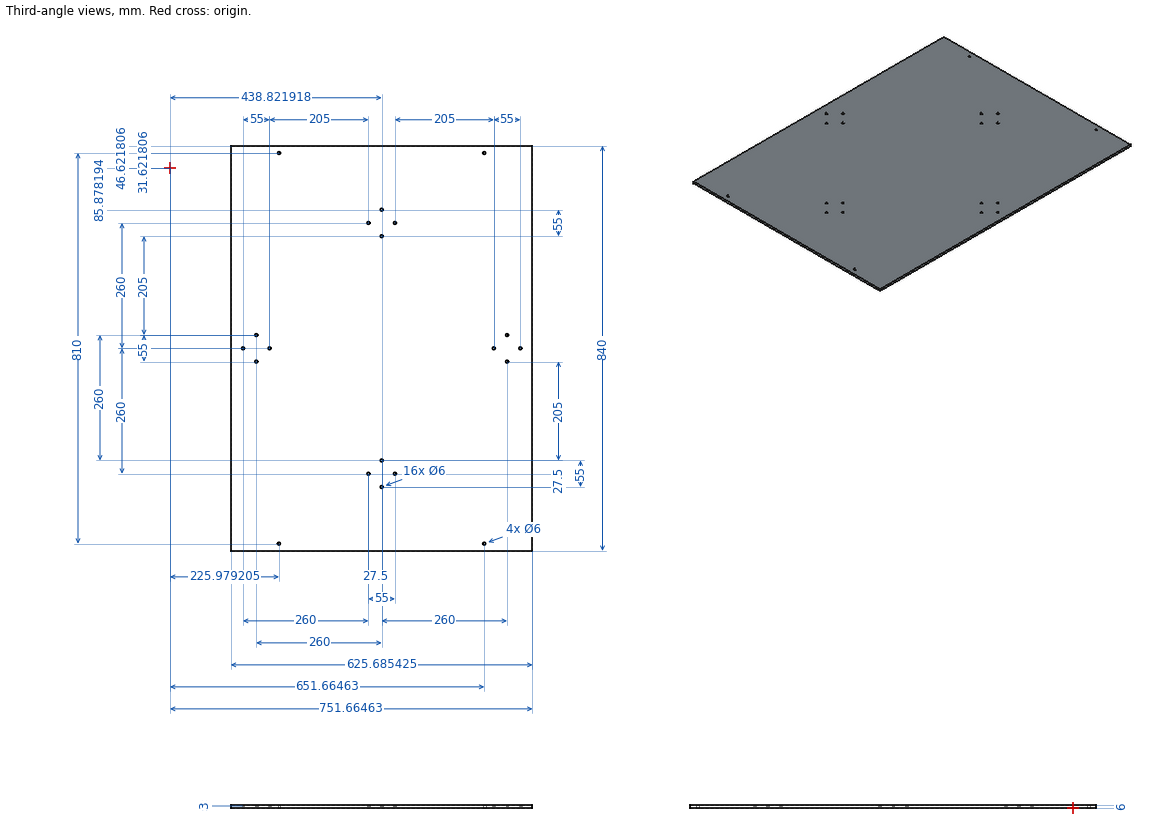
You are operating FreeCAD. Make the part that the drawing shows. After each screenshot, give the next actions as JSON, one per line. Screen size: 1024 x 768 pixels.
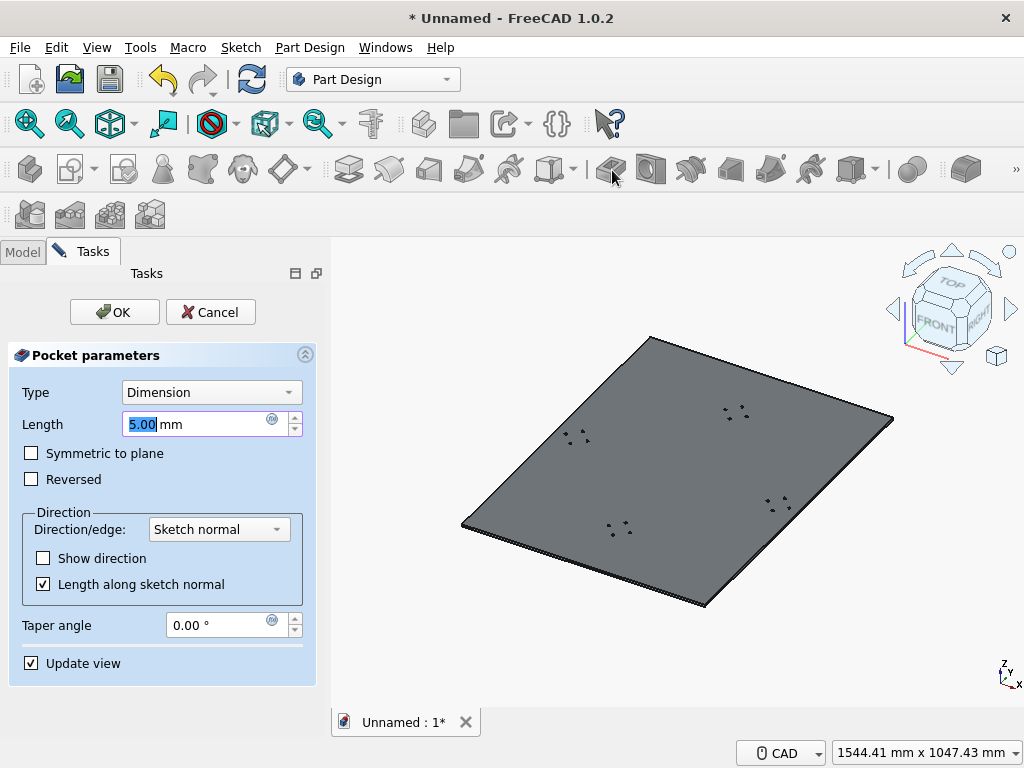
{"action": "type", "text": "3"}
{"action": "key", "text": "Tab"}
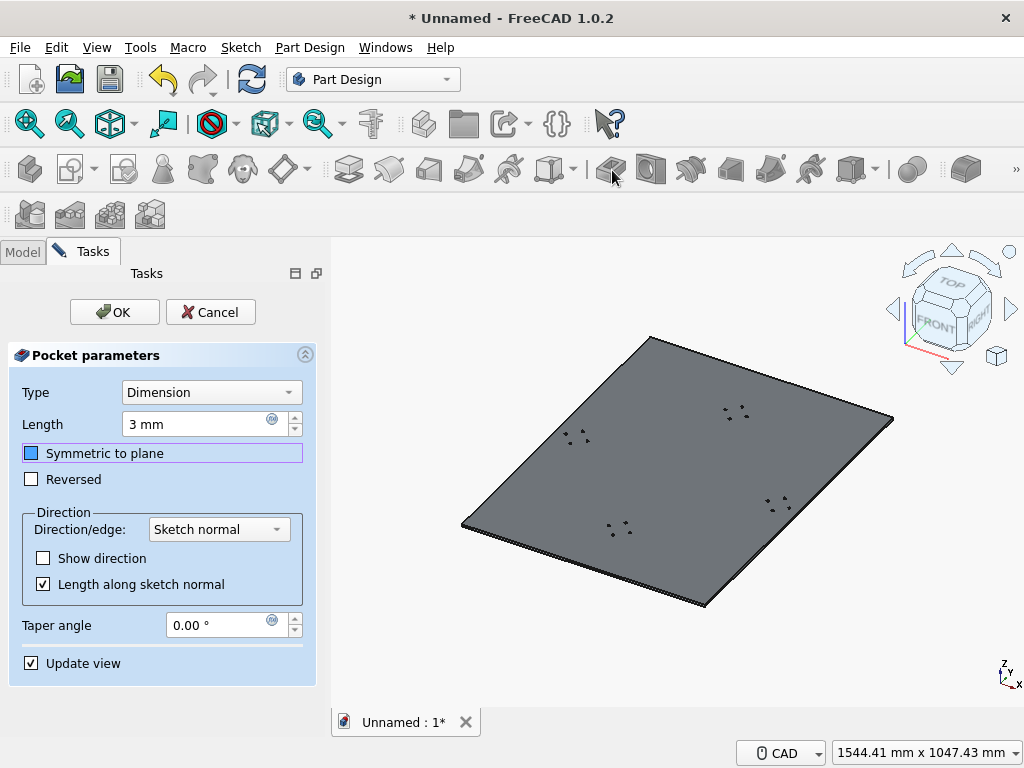
{"action": "left_click", "coordinate": [115, 312]}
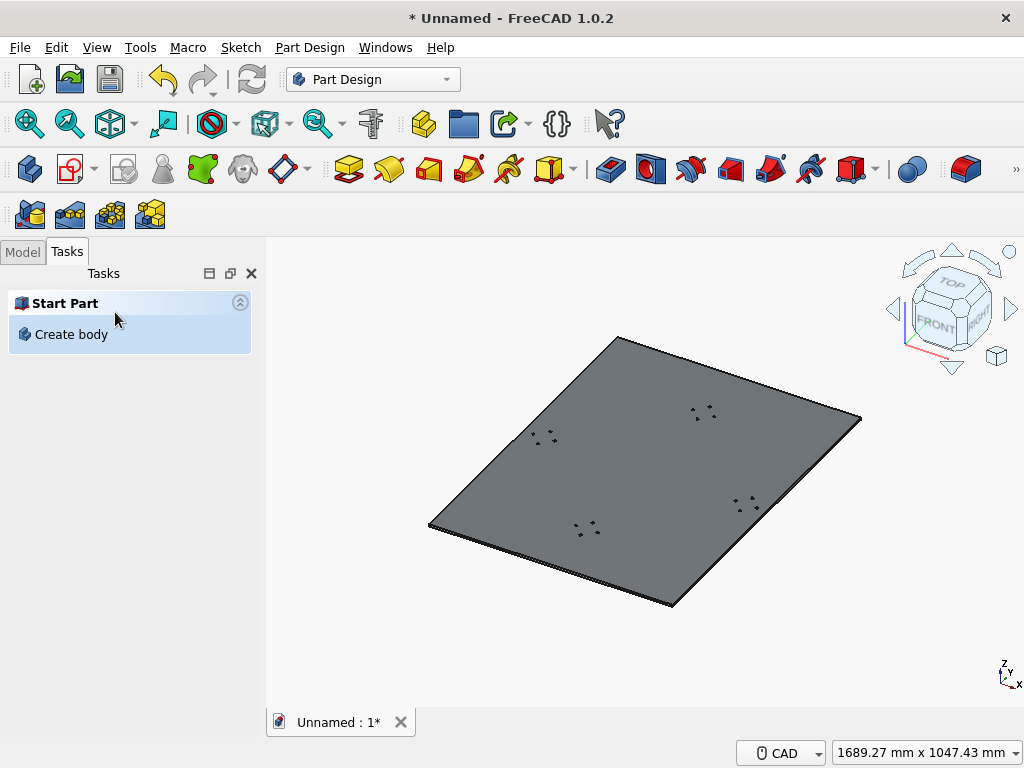
{"action": "left_click", "coordinate": [645, 470]}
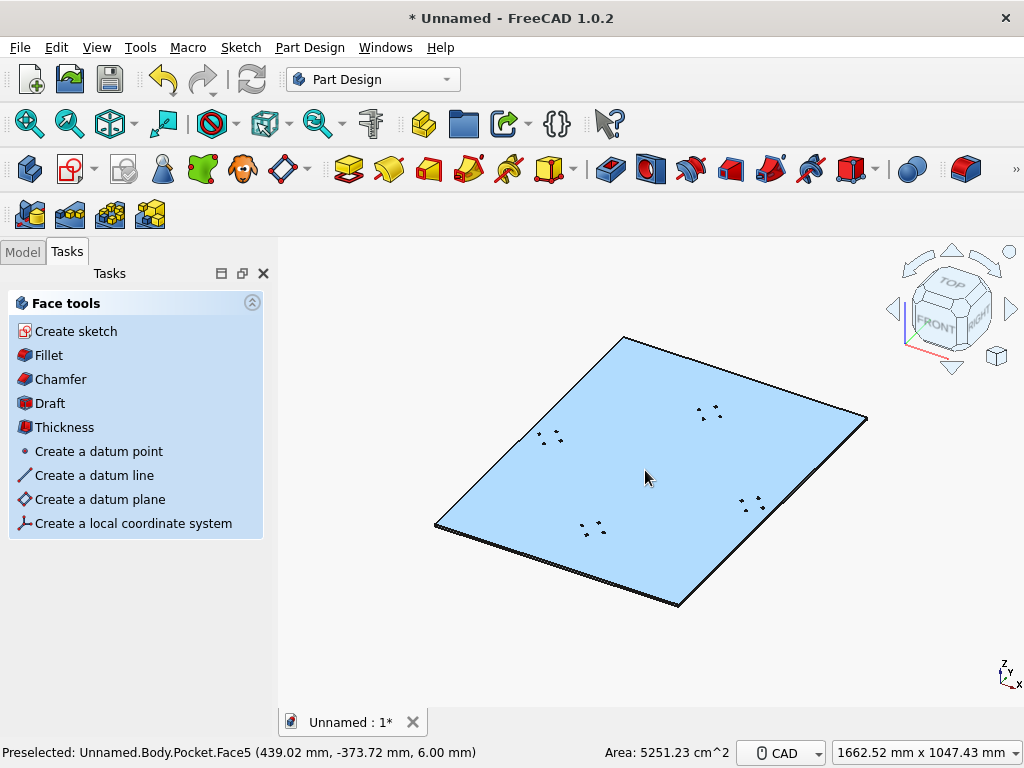
{"action": "left_click", "coordinate": [70, 170]}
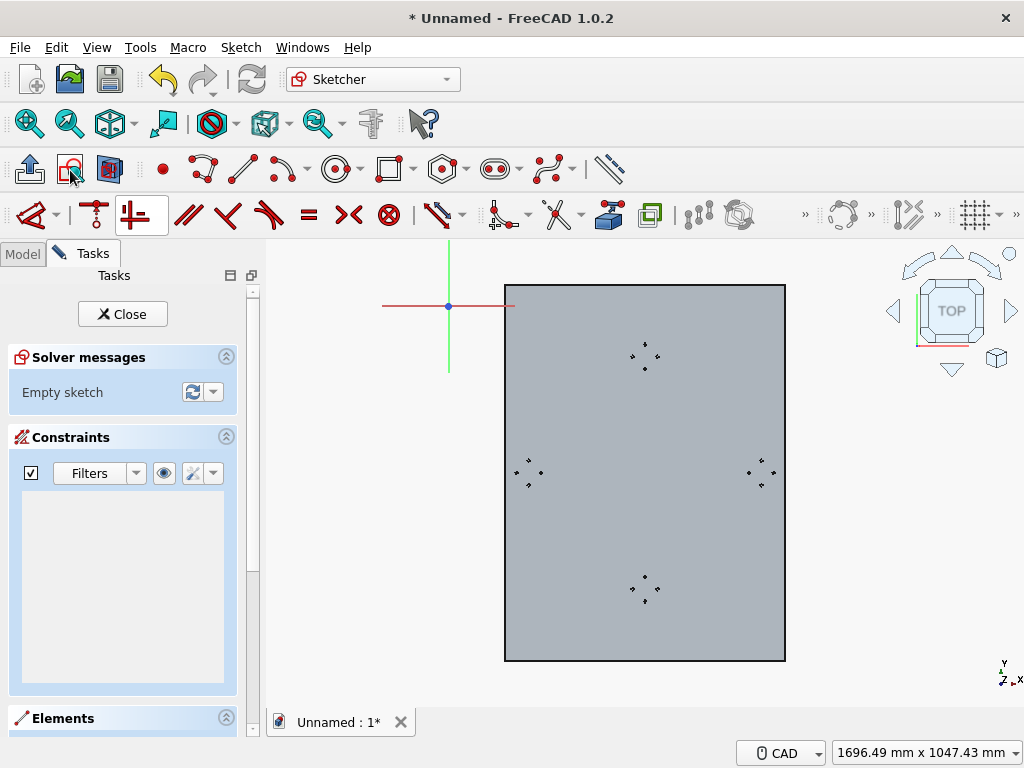
{"action": "scroll", "coordinate": [492, 473], "scroll_direction": "down", "scroll_amount": 1}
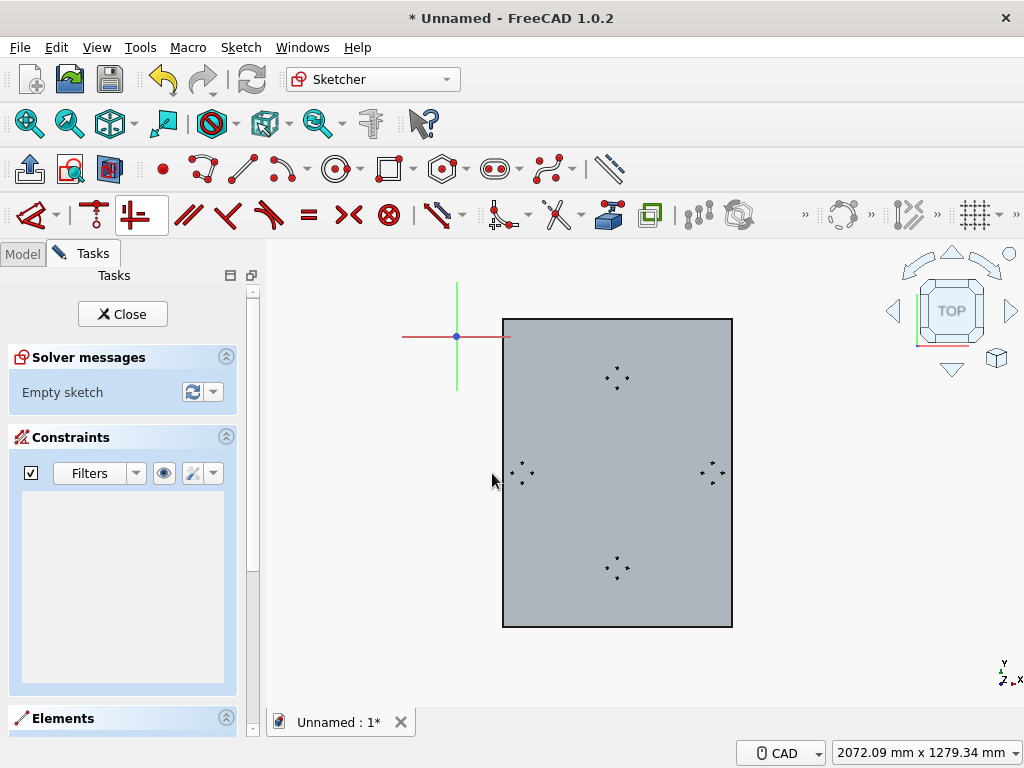
{"action": "left_click", "coordinate": [336, 170]}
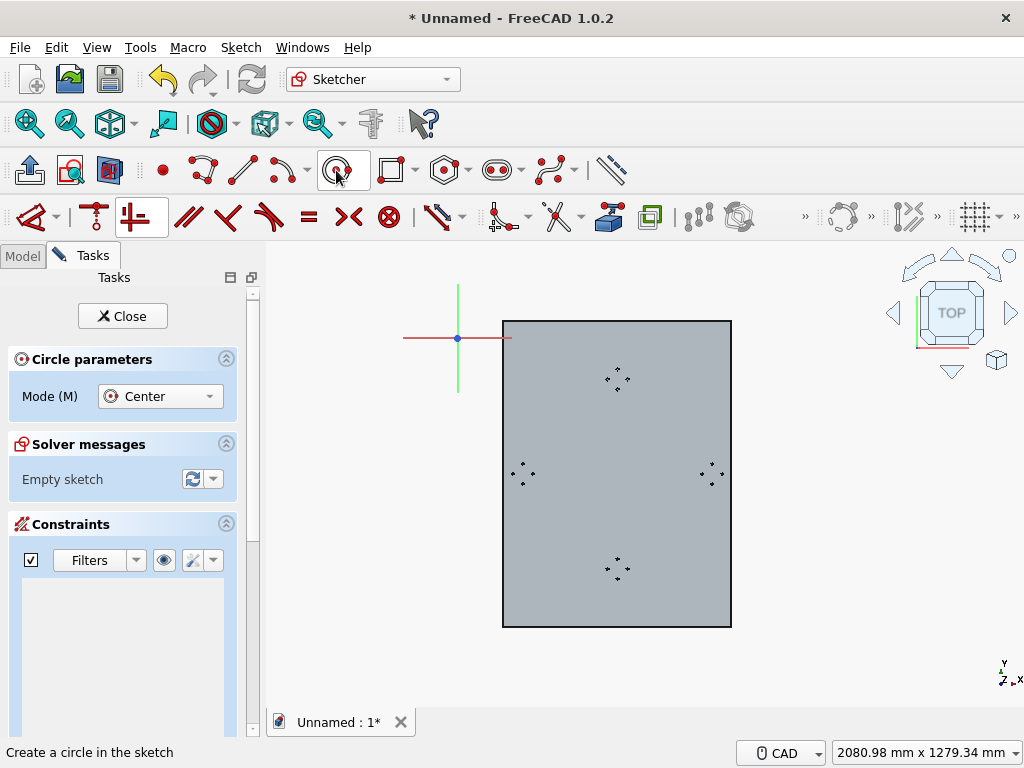
{"action": "scroll", "coordinate": [695, 622], "scroll_direction": "up", "scroll_amount": 16}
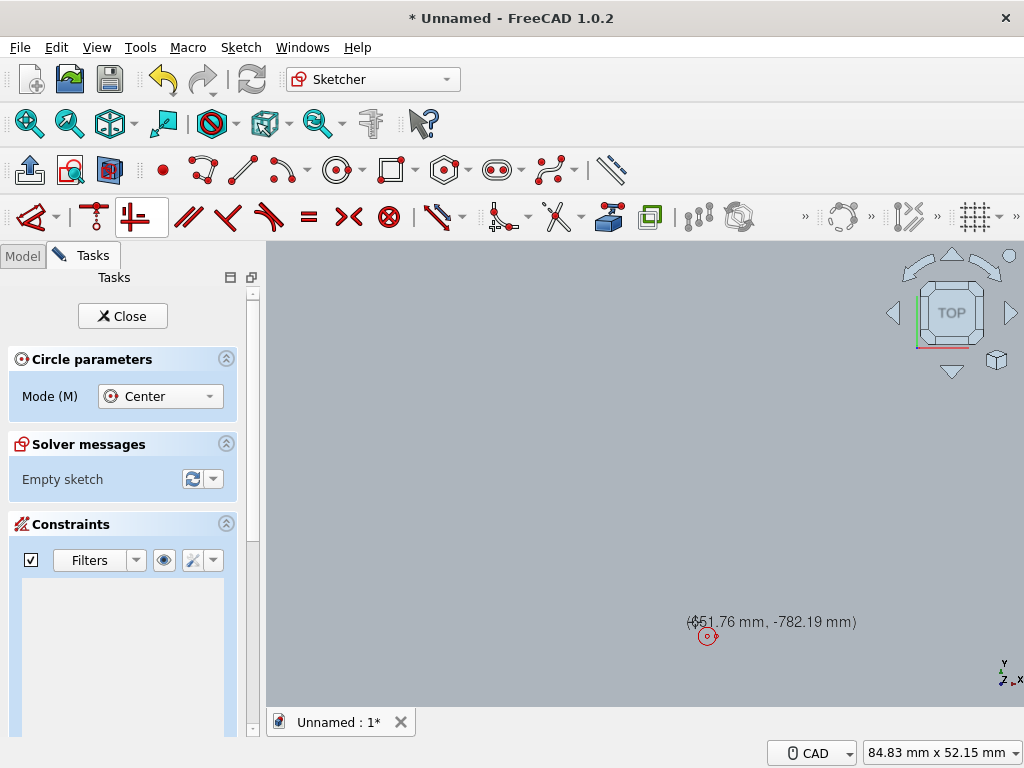
{"action": "scroll", "coordinate": [695, 623], "scroll_direction": "down", "scroll_amount": 16}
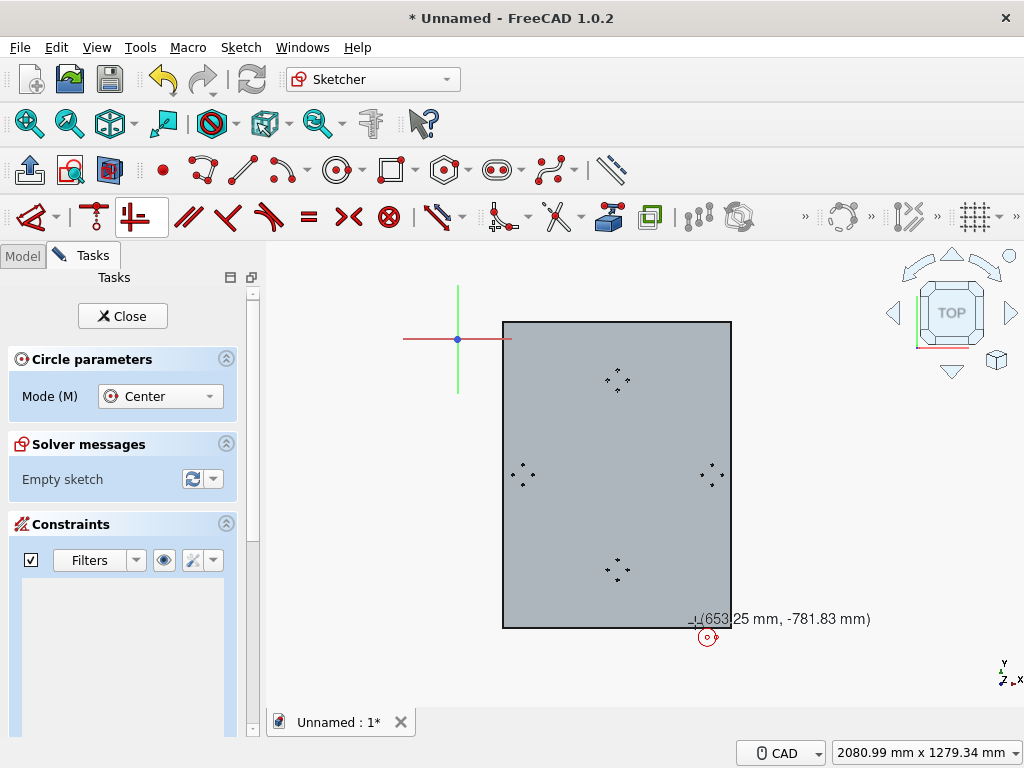
{"action": "left_click", "coordinate": [695, 623]}
{"action": "mouse_move", "coordinate": [696, 622]}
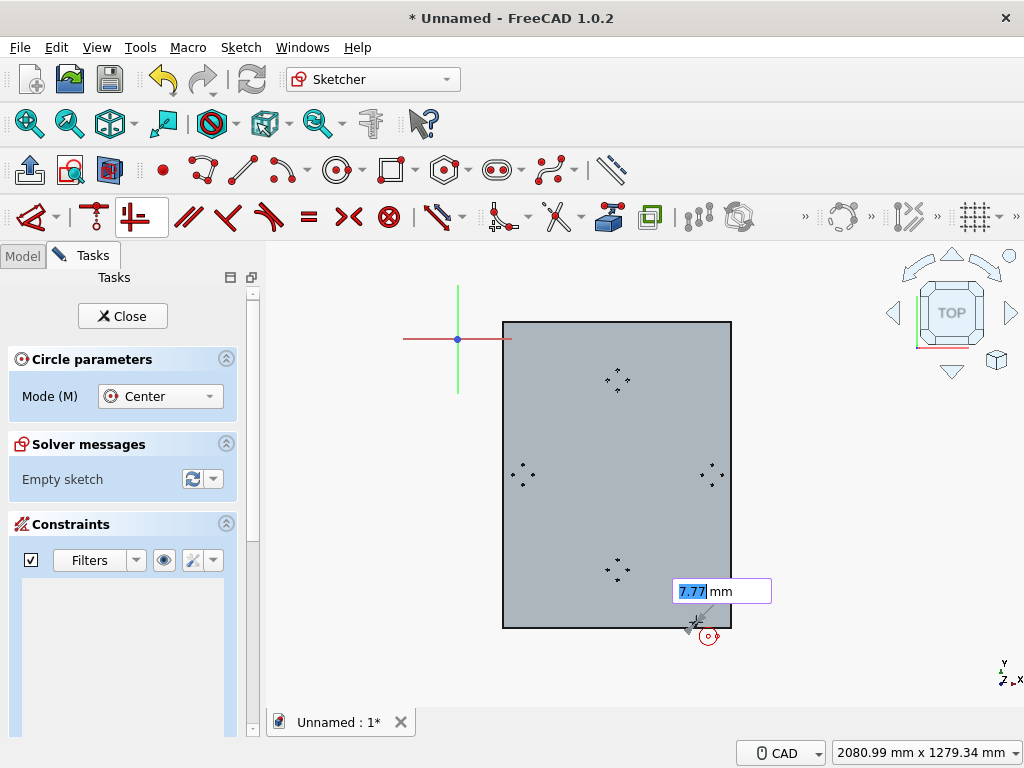
{"action": "type", "text": "6"}
{"action": "key", "text": "Return"}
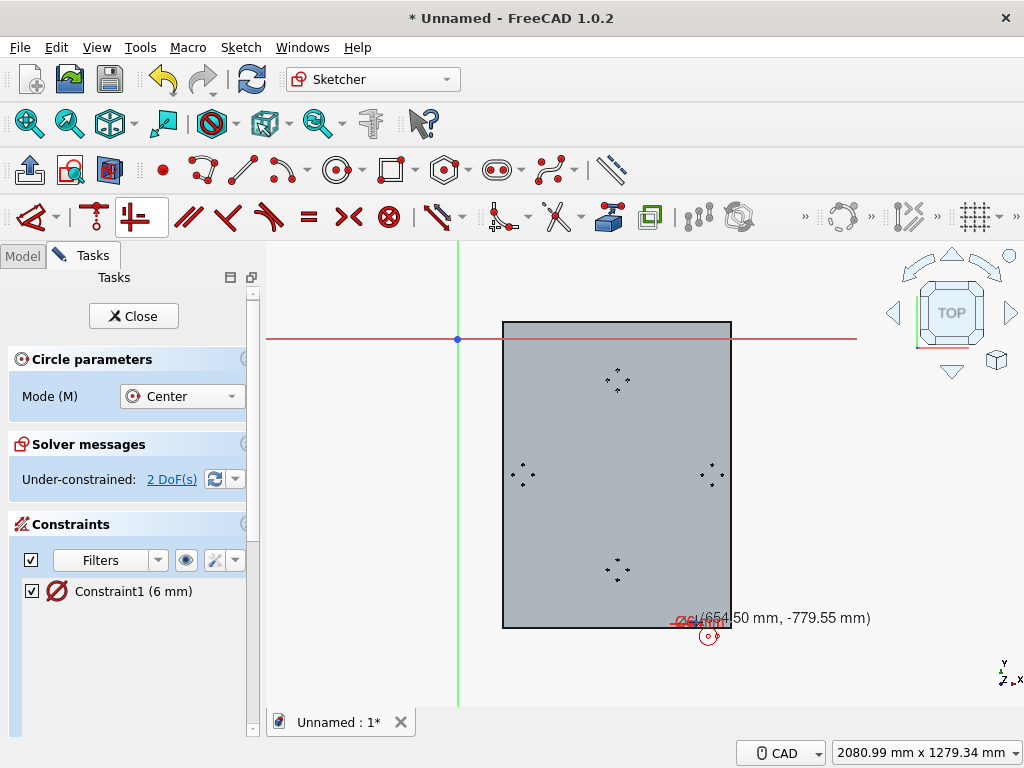
{"action": "scroll", "coordinate": [540, 623], "scroll_direction": "up", "scroll_amount": 16}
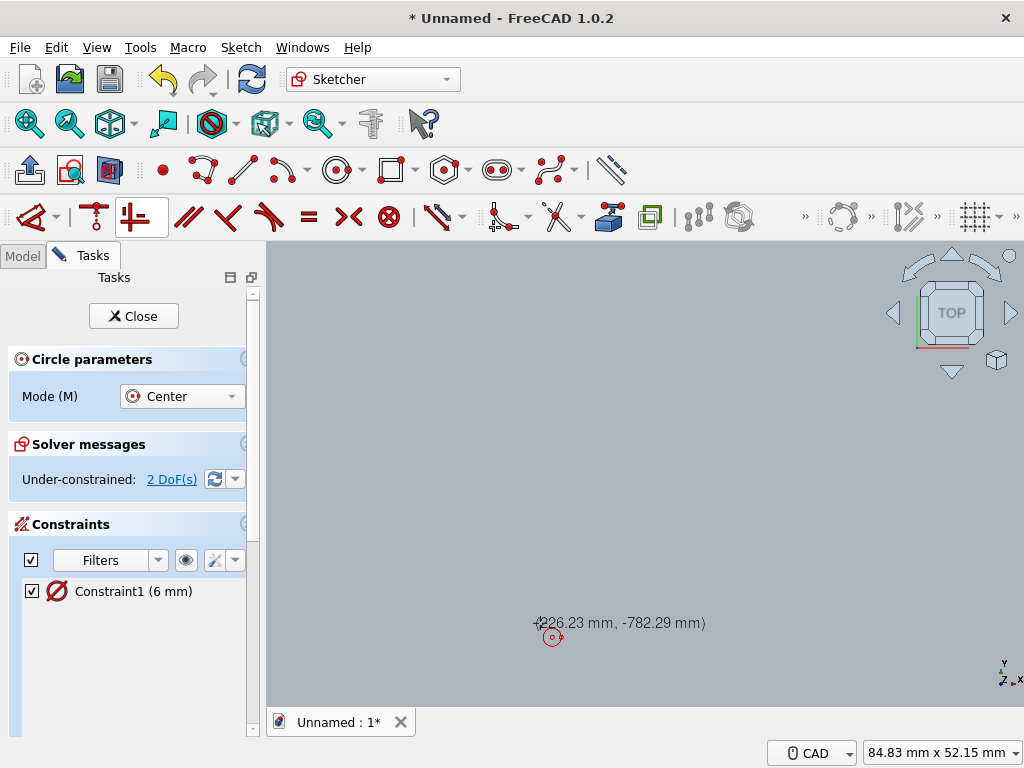
{"action": "scroll", "coordinate": [540, 623], "scroll_direction": "down", "scroll_amount": 16}